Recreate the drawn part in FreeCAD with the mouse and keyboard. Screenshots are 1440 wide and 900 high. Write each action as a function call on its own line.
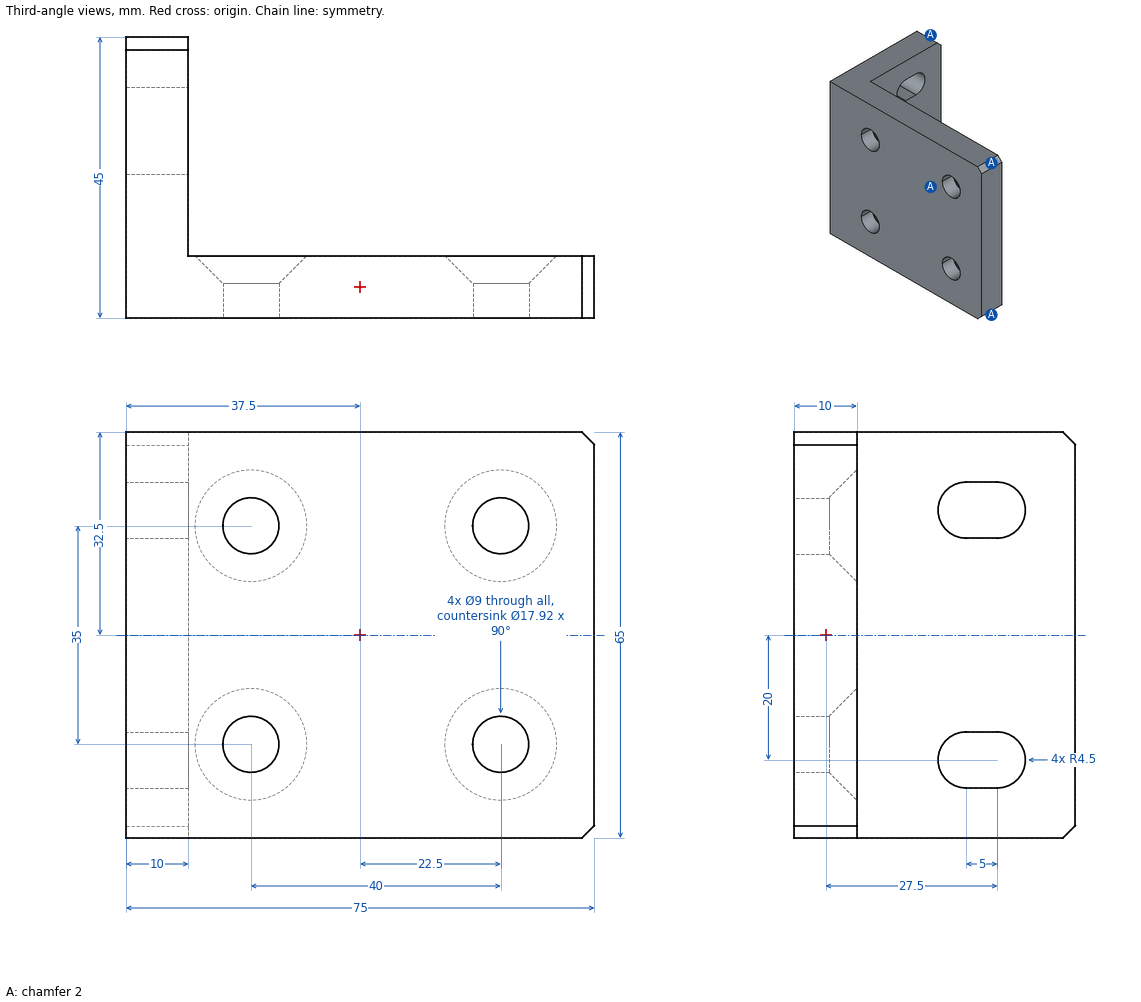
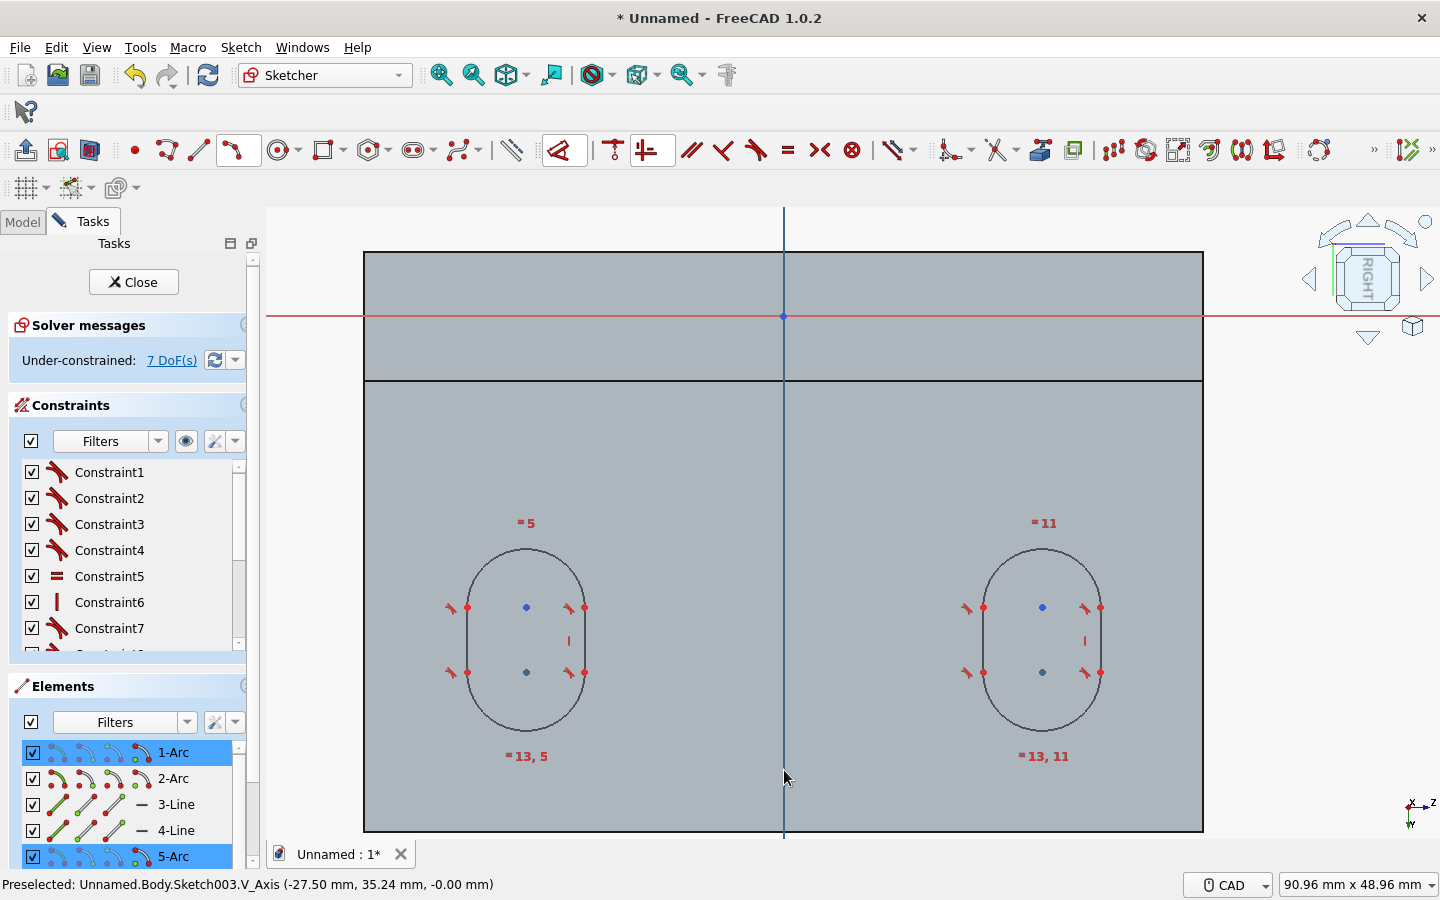
key(s)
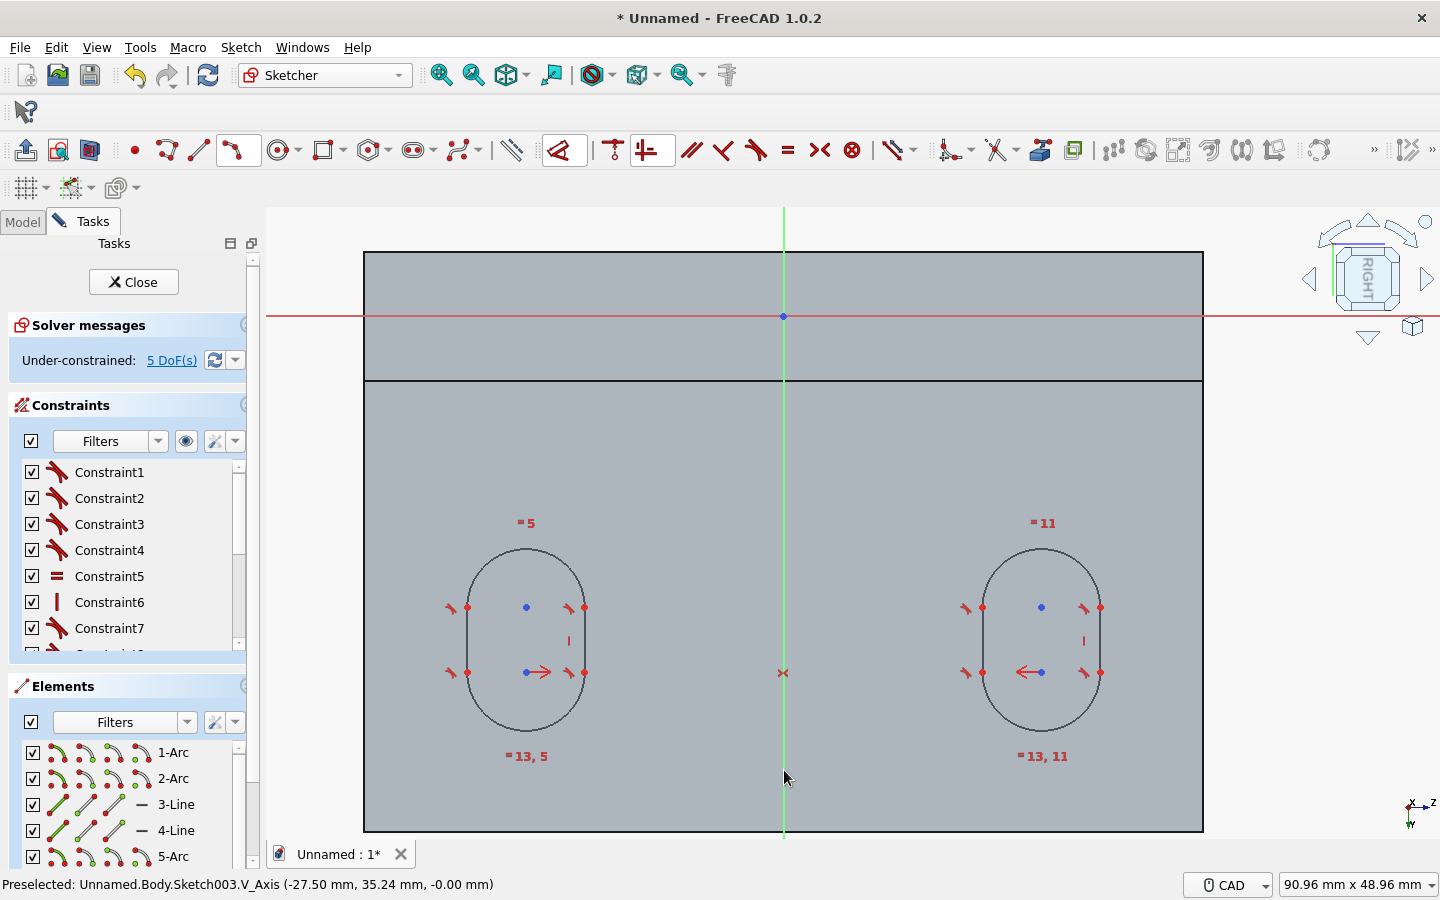
key(d)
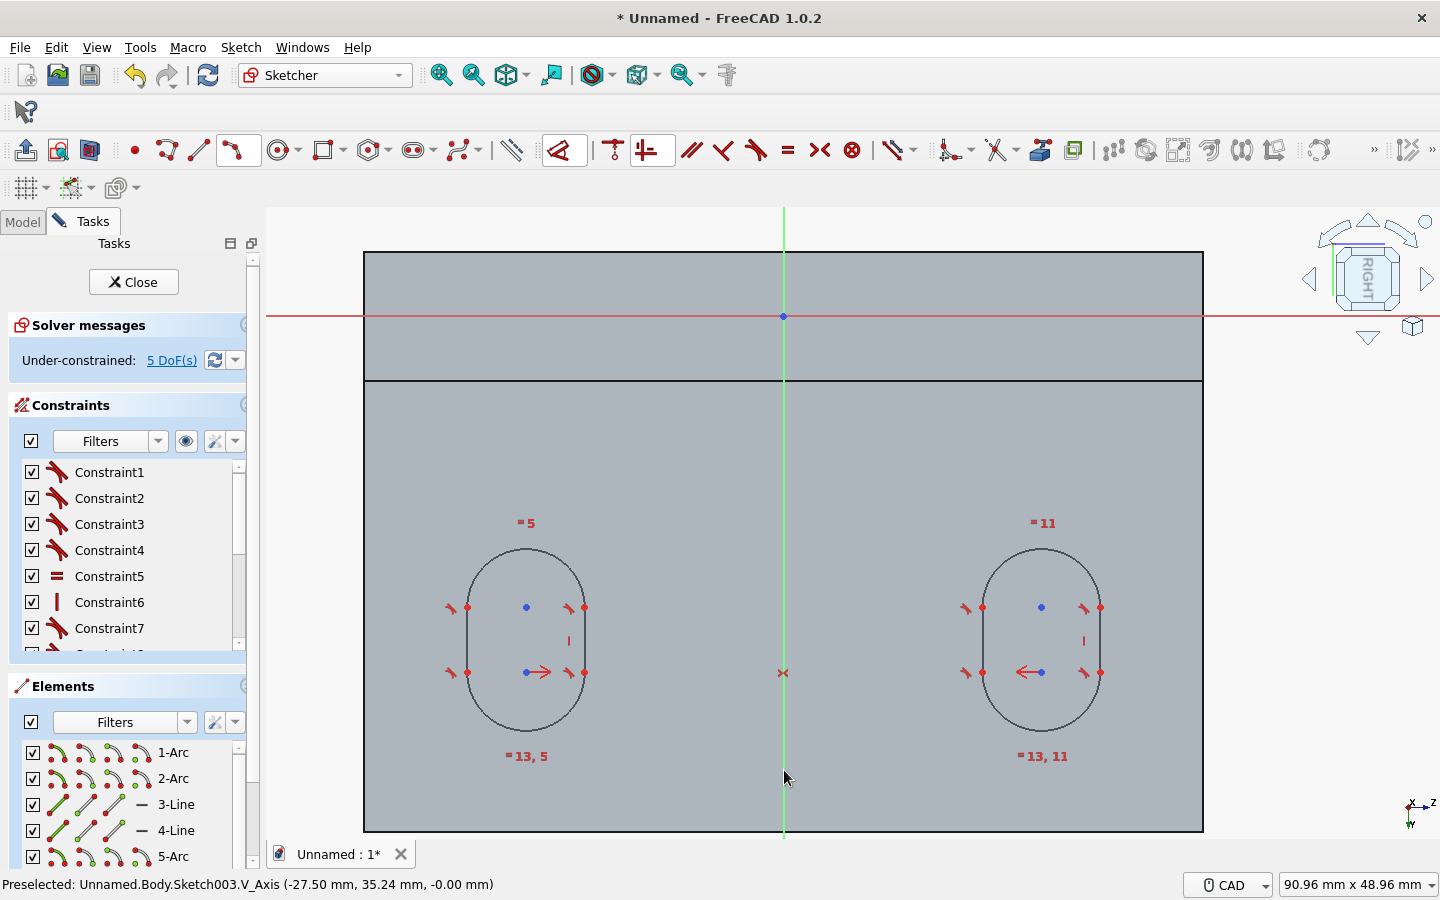
click(491, 720)
click(472, 746)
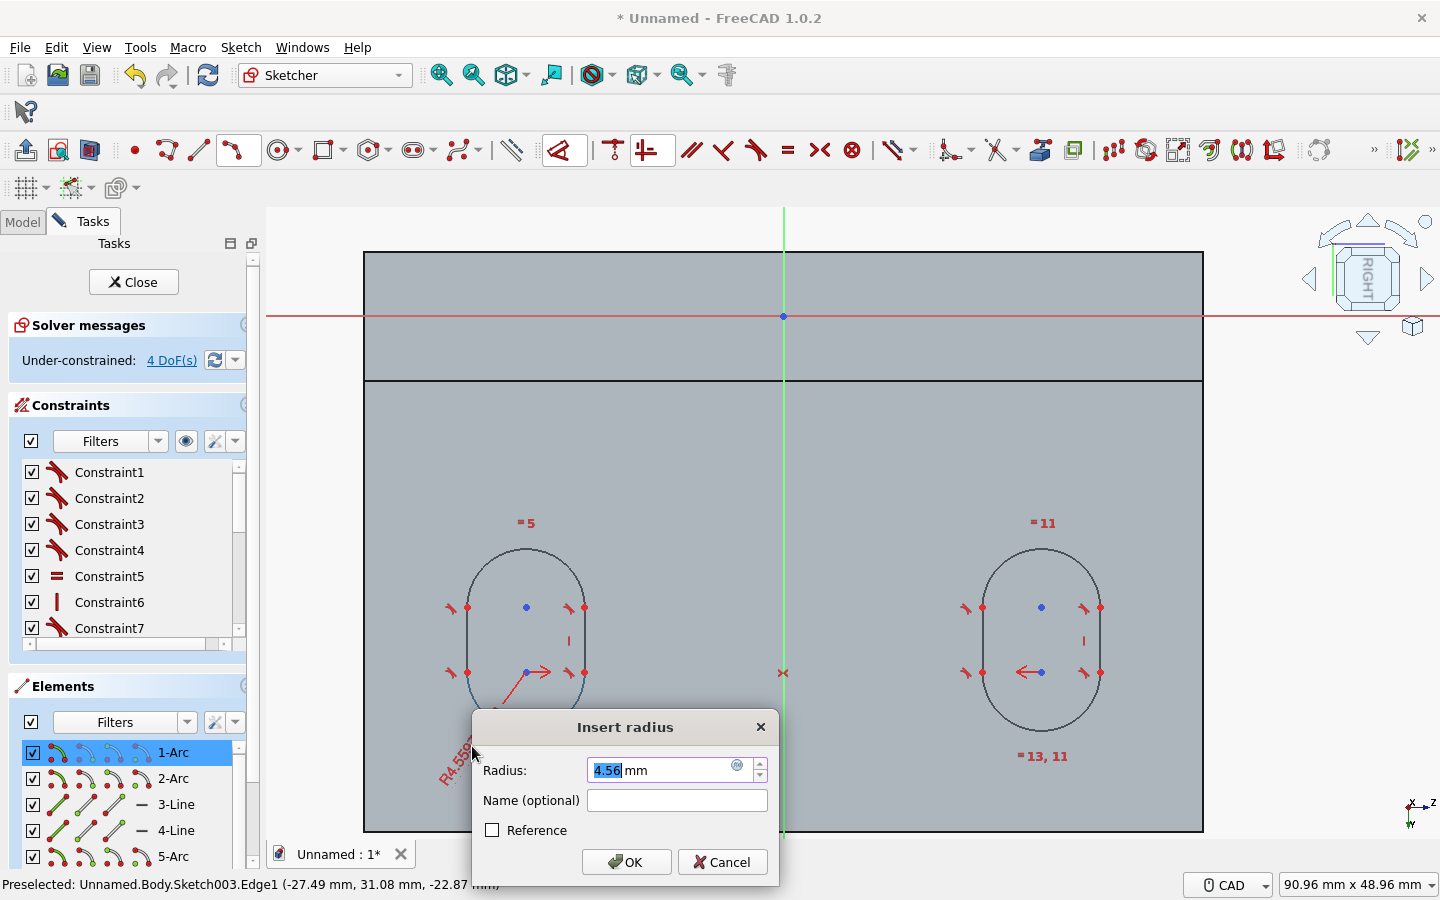
text(4.5)
key(Return)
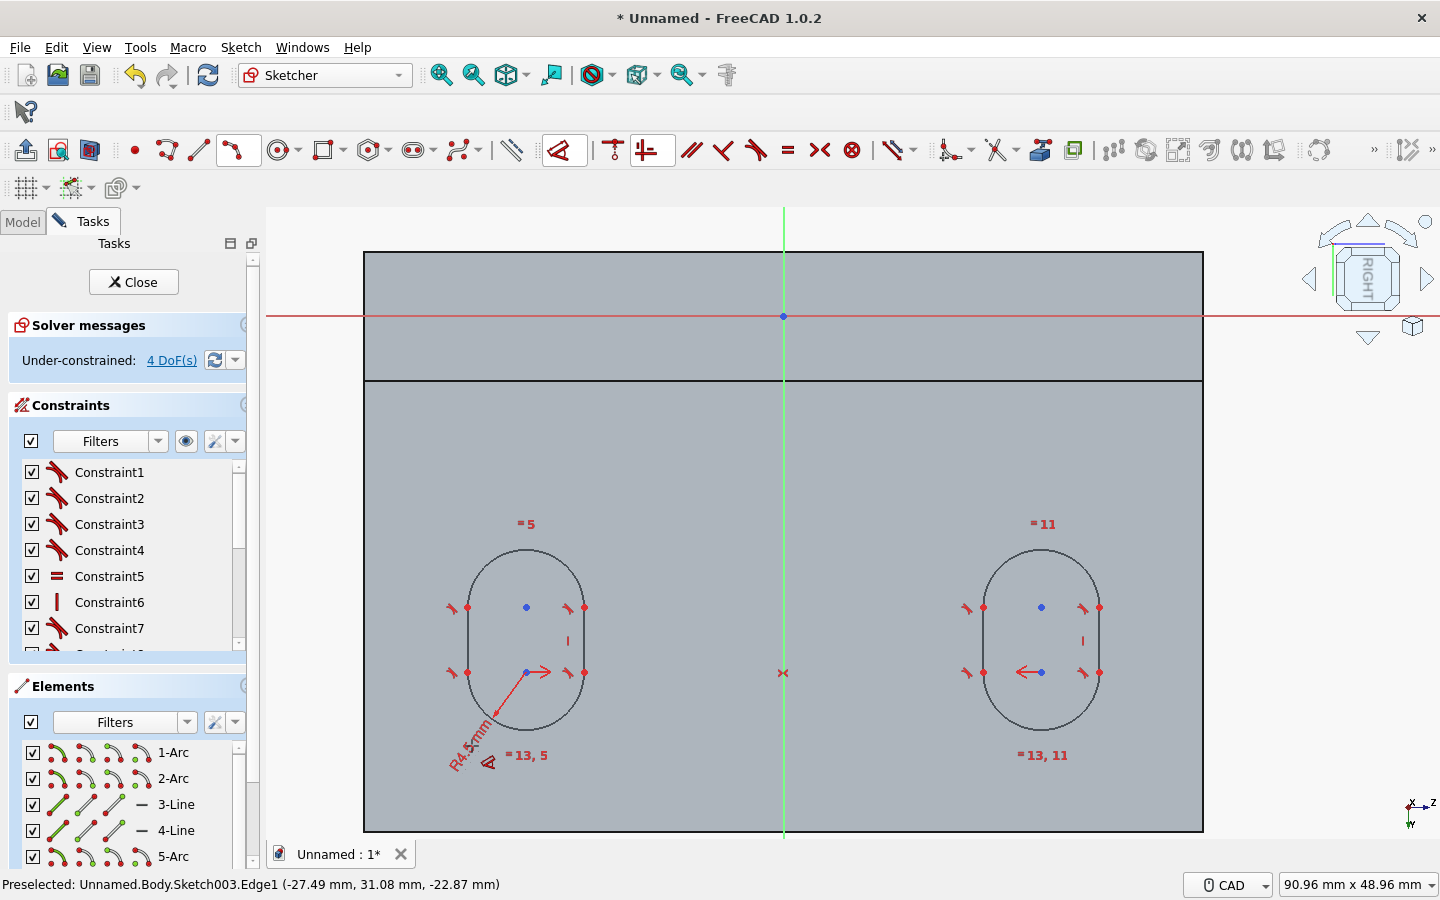
click(468, 653)
click(434, 640)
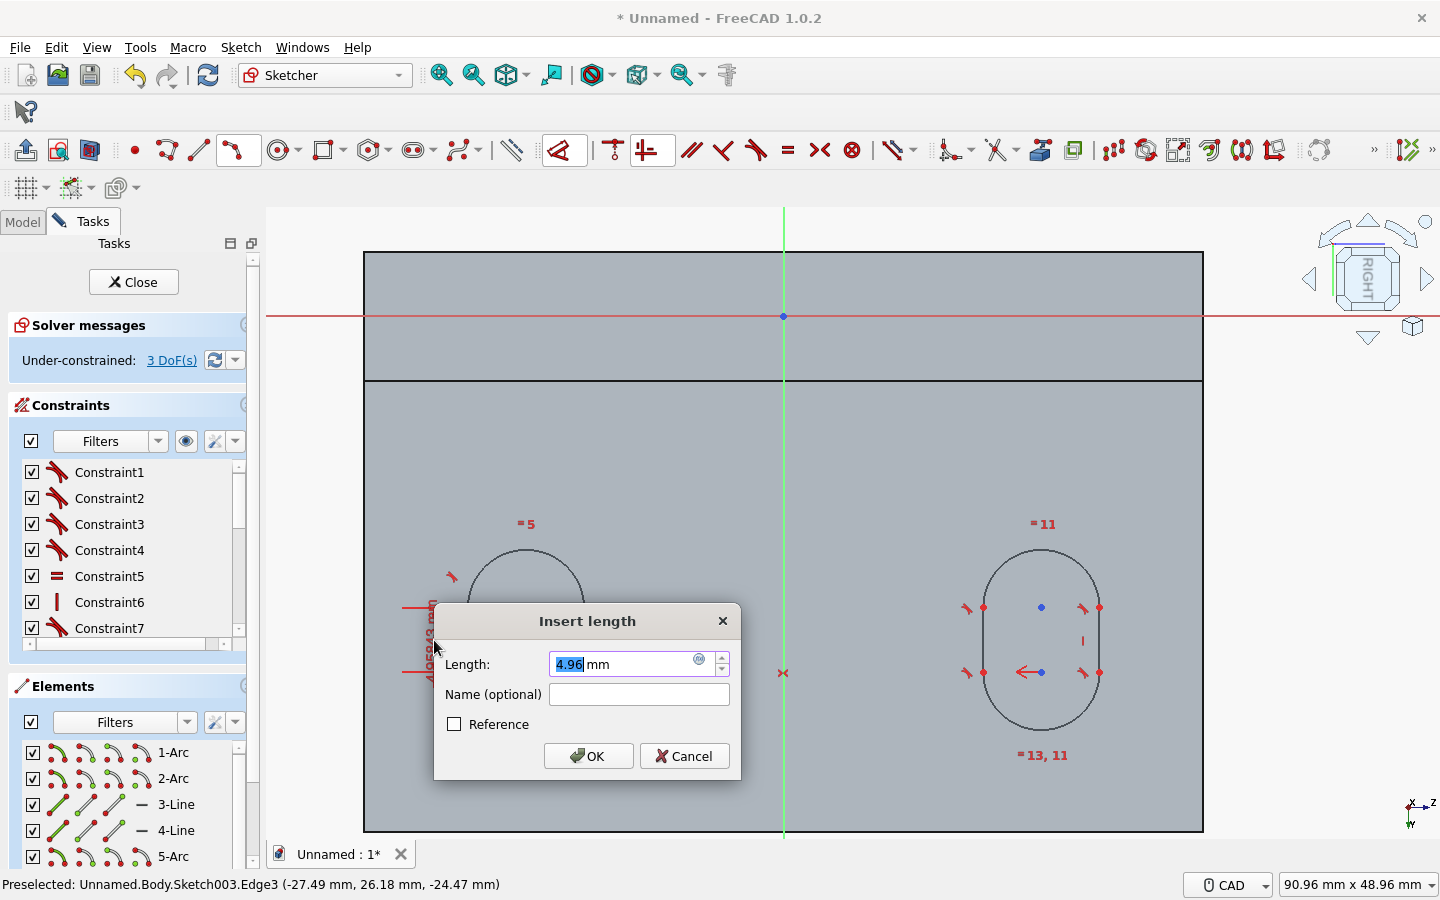
text(5)
key(Return)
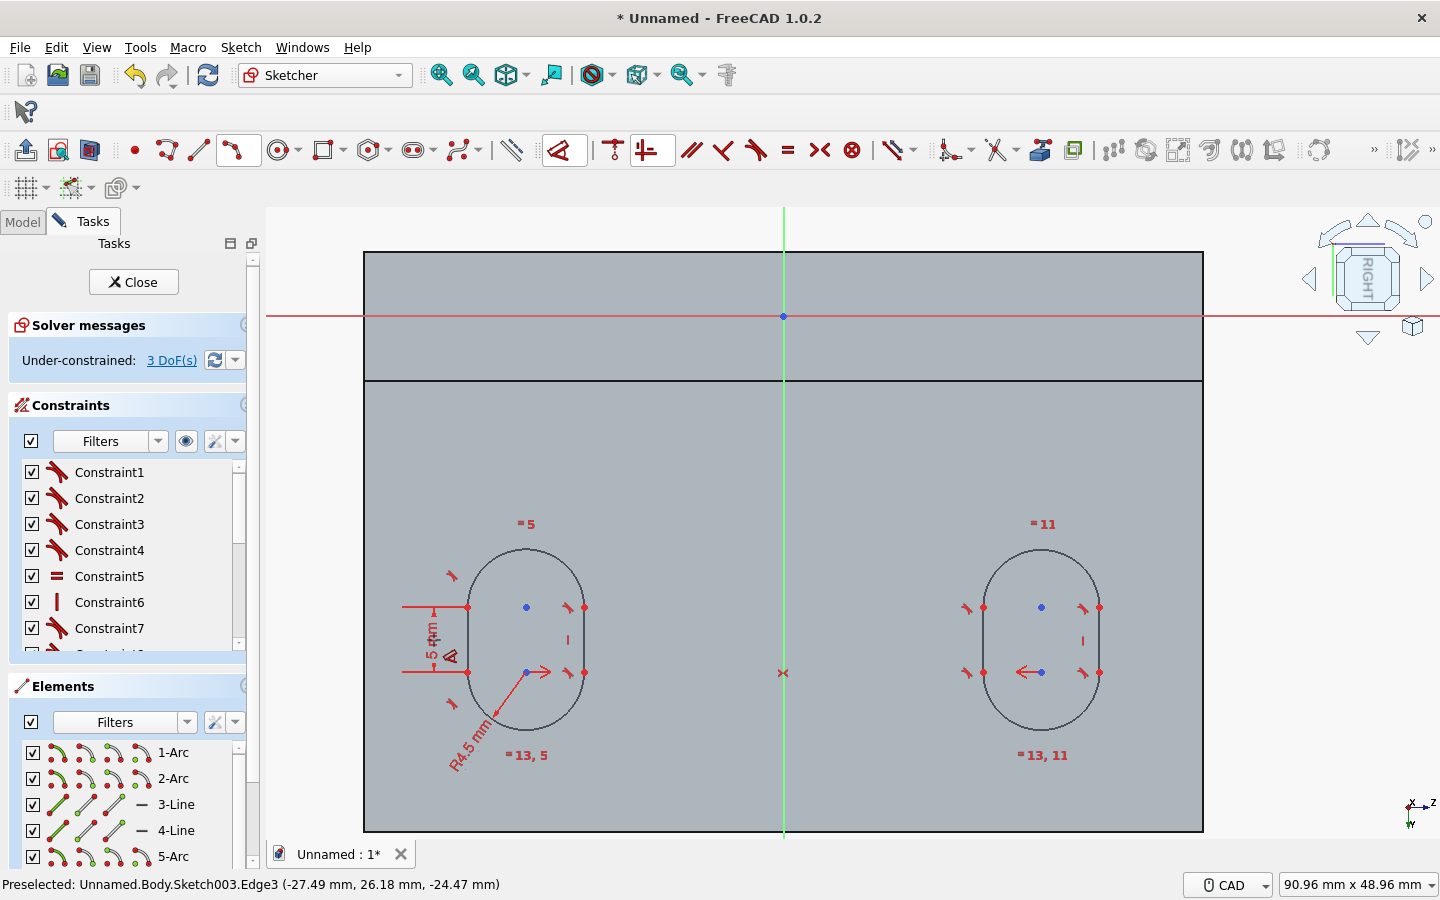
click(983, 653)
click(1017, 640)